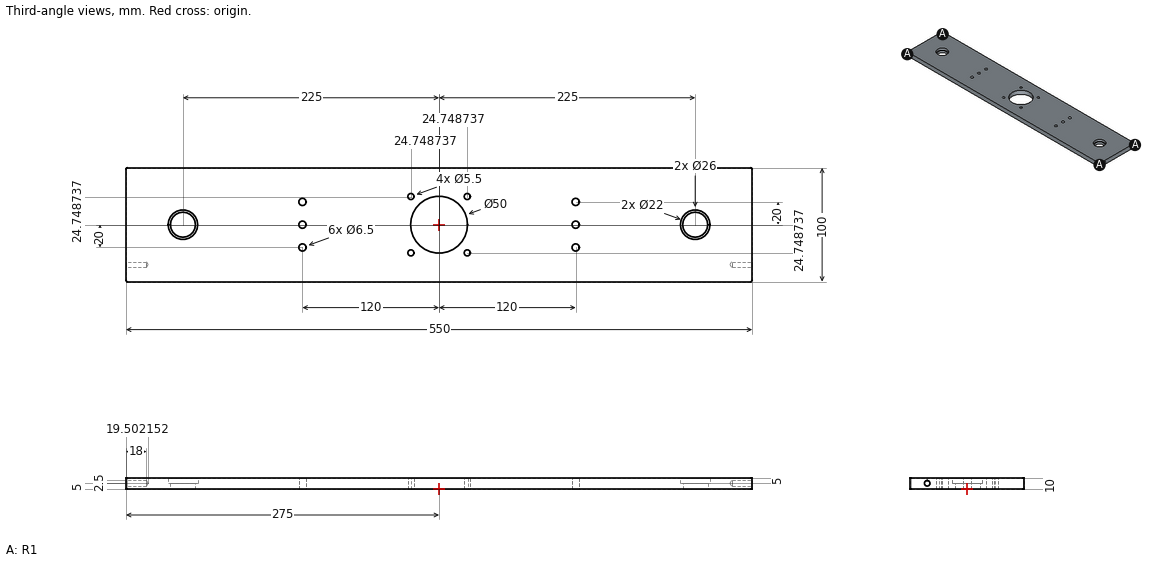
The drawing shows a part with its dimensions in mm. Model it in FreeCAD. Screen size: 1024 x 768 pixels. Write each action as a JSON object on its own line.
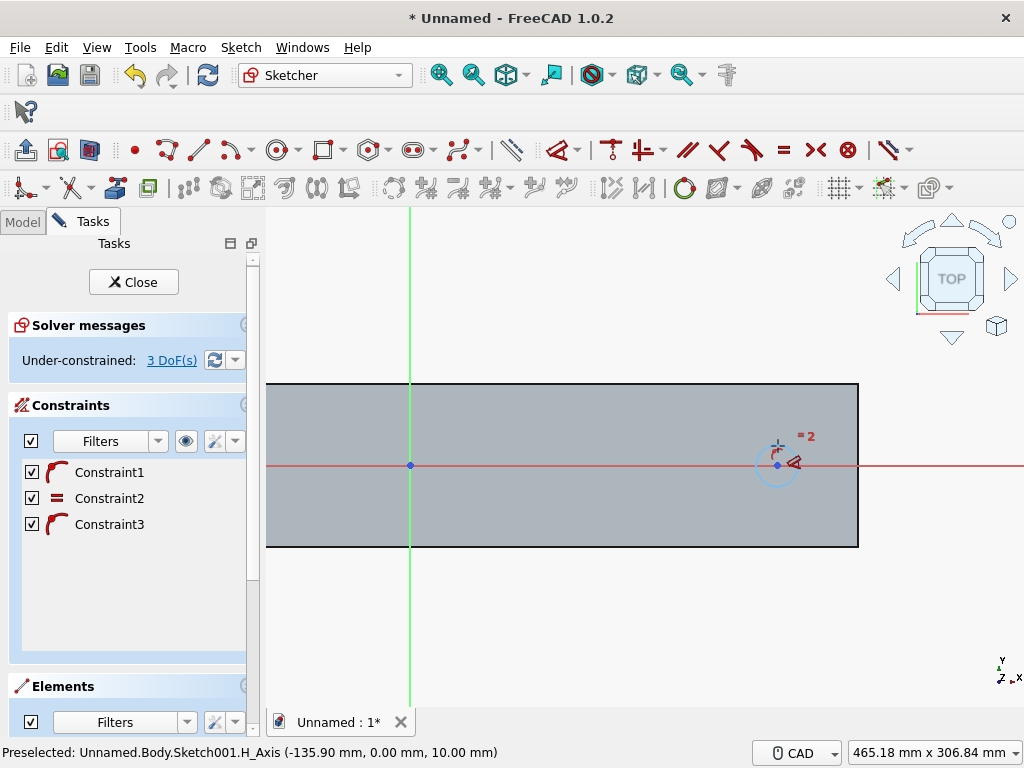
{"action": "left_click", "coordinate": [778, 445]}
{"action": "left_click", "coordinate": [779, 413]}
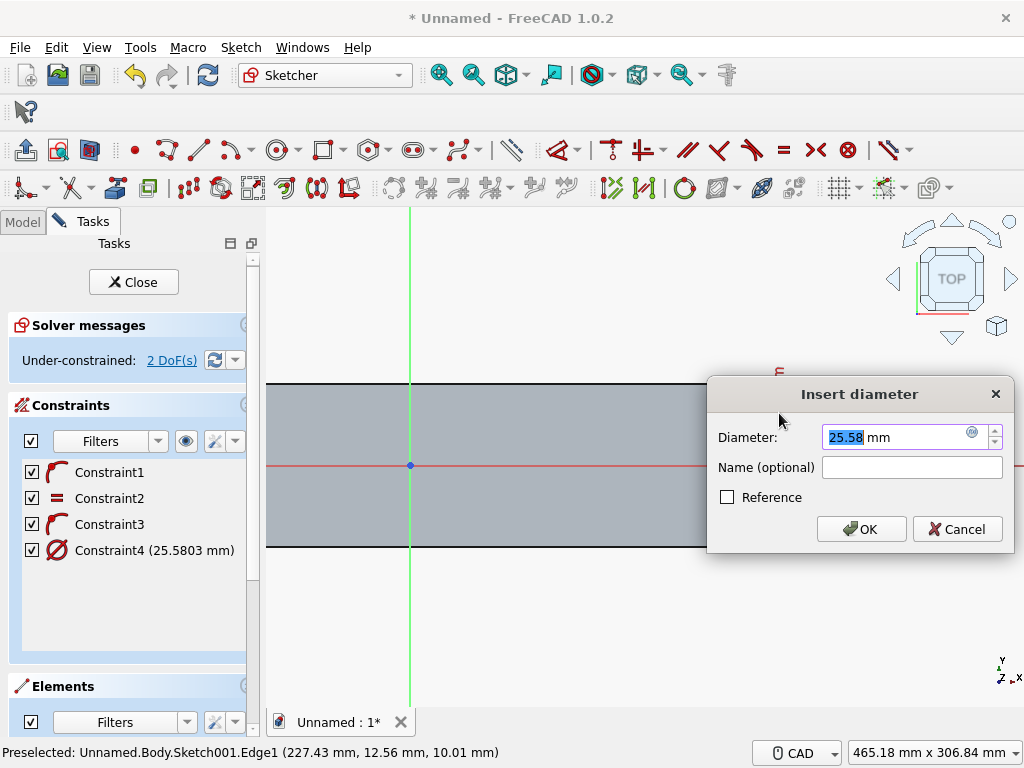
{"action": "type", "text": "26"}
{"action": "key", "text": "Return"}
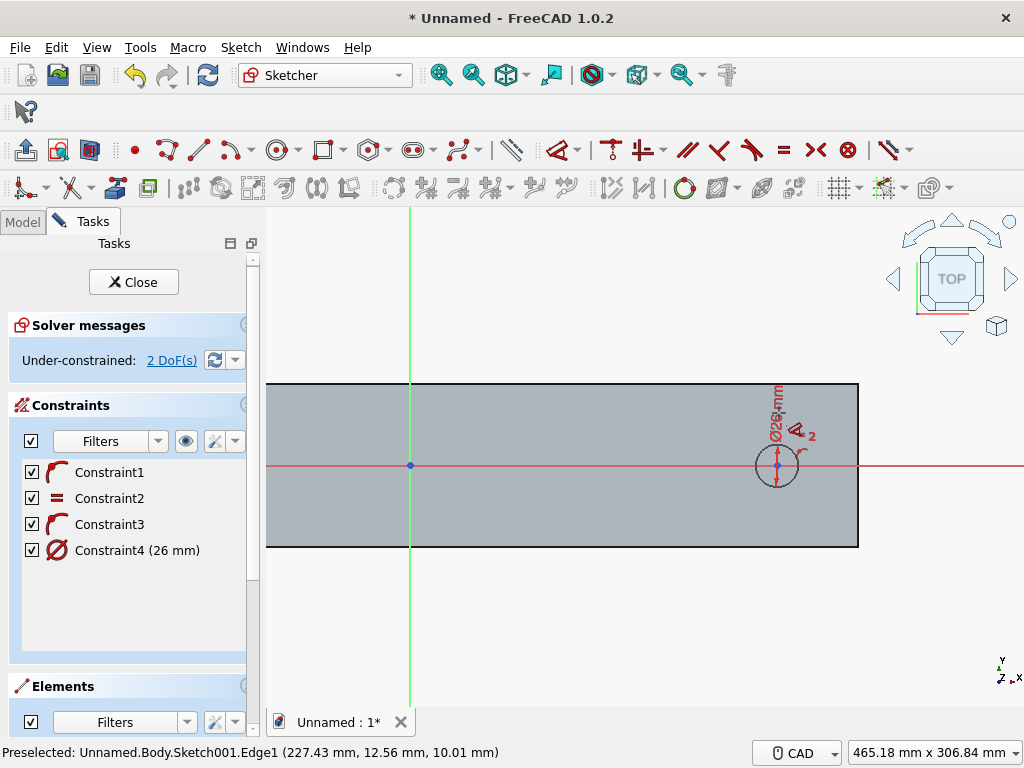
{"action": "left_click", "coordinate": [777, 466]}
{"action": "left_click", "coordinate": [594, 500]}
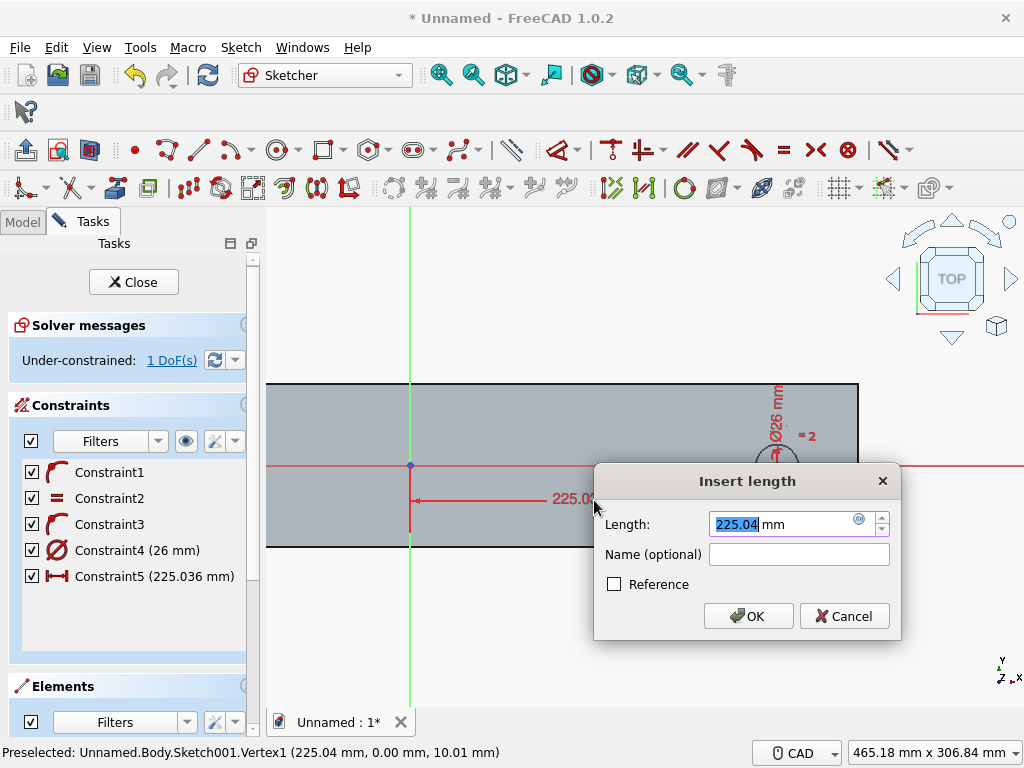
{"action": "type", "text": "225"}
{"action": "key", "text": "Return"}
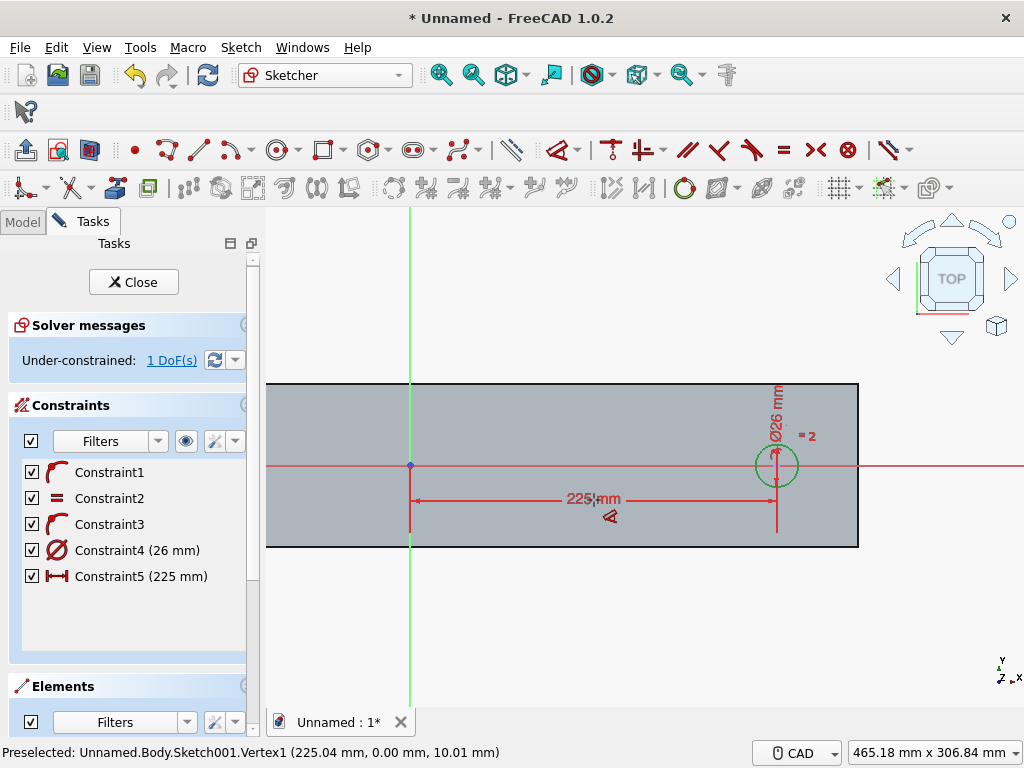
{"action": "scroll", "coordinate": [779, 446], "scroll_direction": "down", "scroll_amount": 3}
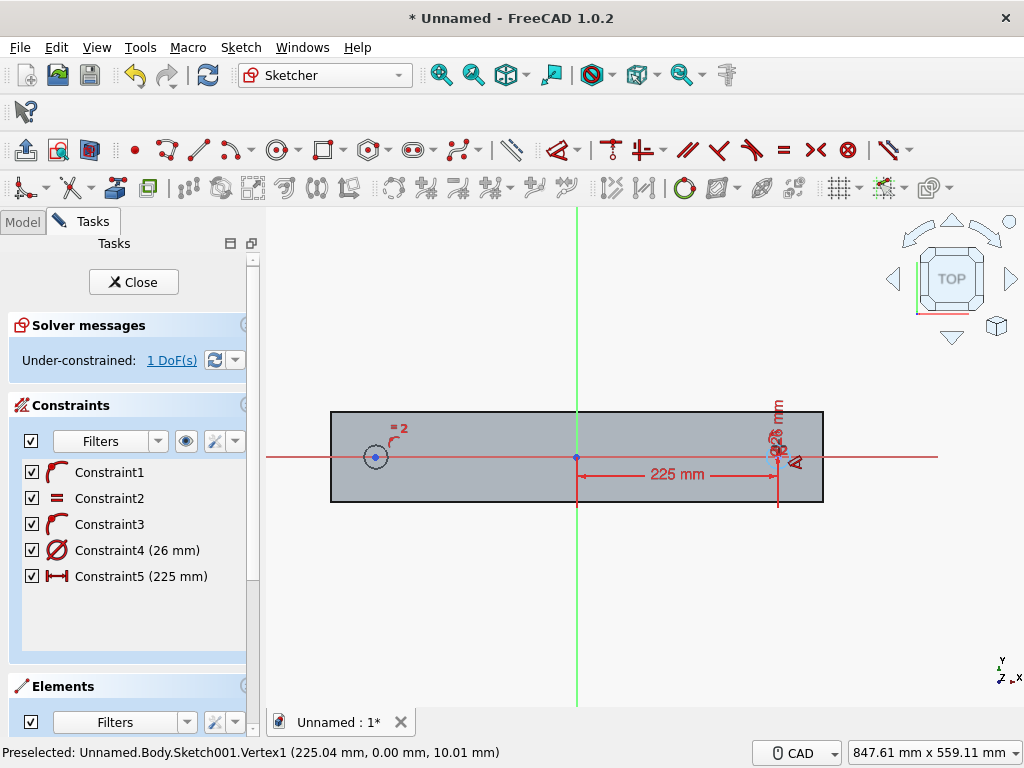
{"action": "left_click", "coordinate": [376, 457]}
{"action": "left_click", "coordinate": [476, 491]}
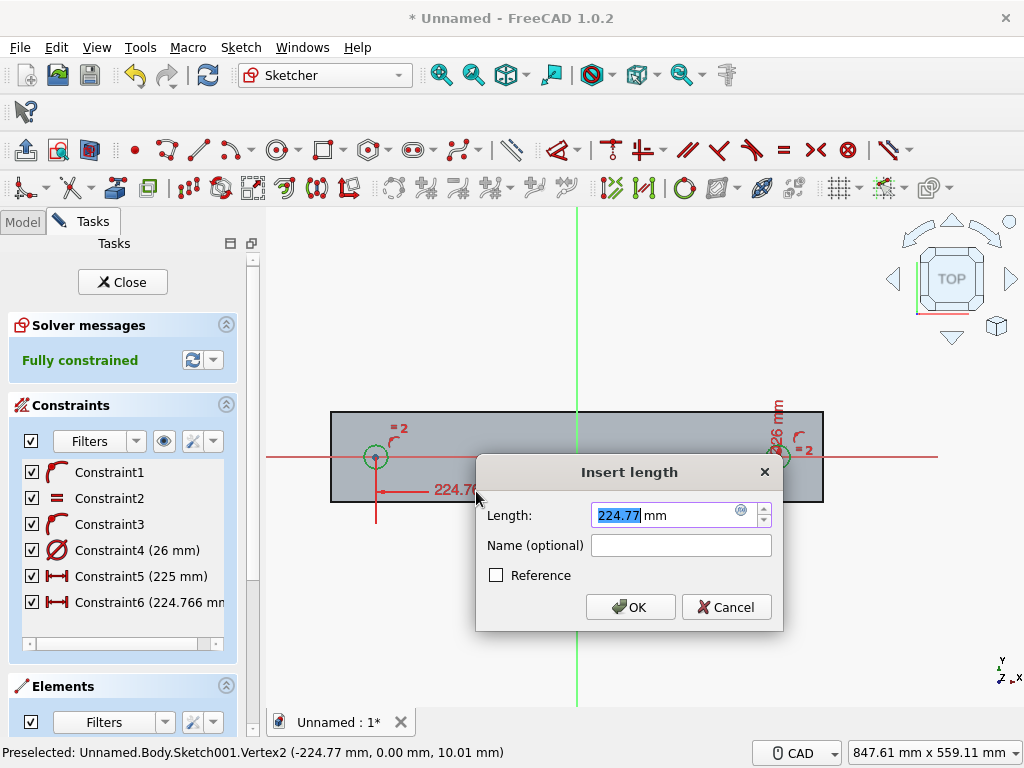
{"action": "type", "text": "225"}
{"action": "key", "text": "Return"}
{"action": "key", "text": "Escape"}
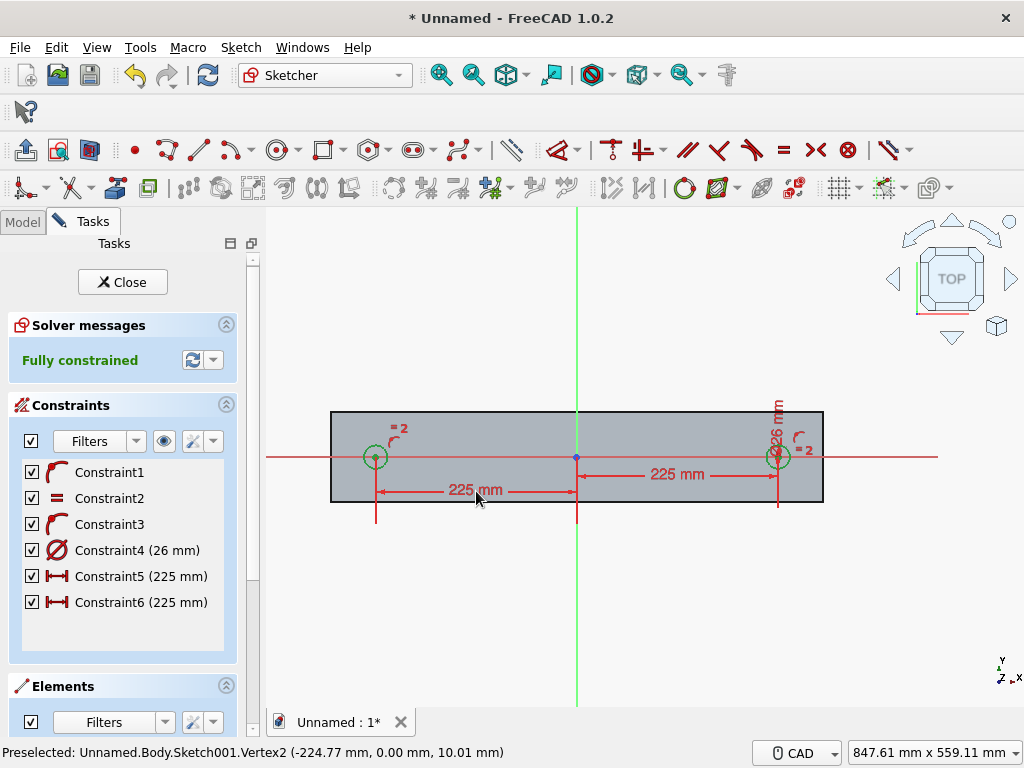
{"action": "left_click", "coordinate": [123, 282]}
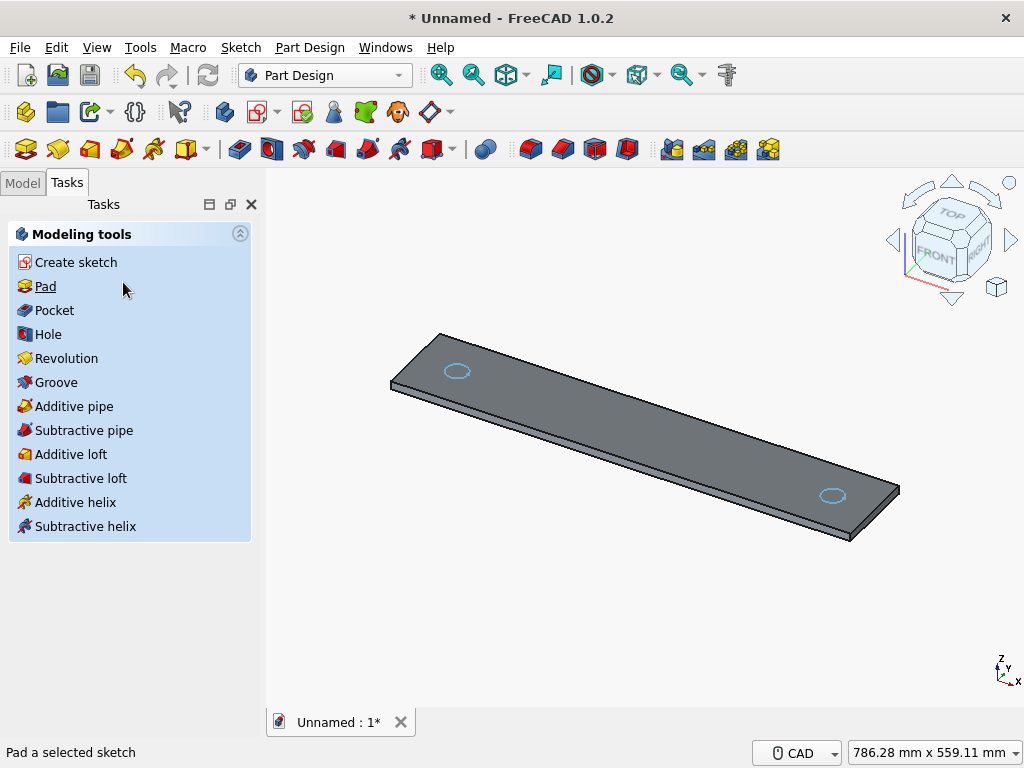
{"action": "left_click", "coordinate": [240, 150]}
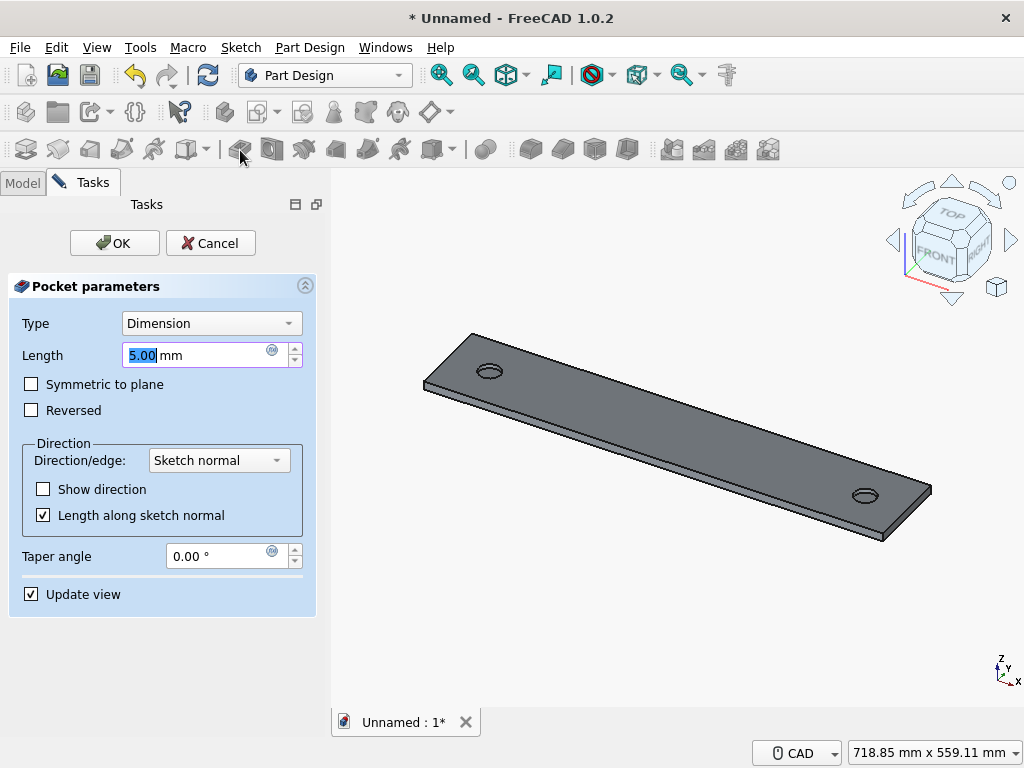
{"action": "type", "text": "5"}
{"action": "key", "text": "Tab"}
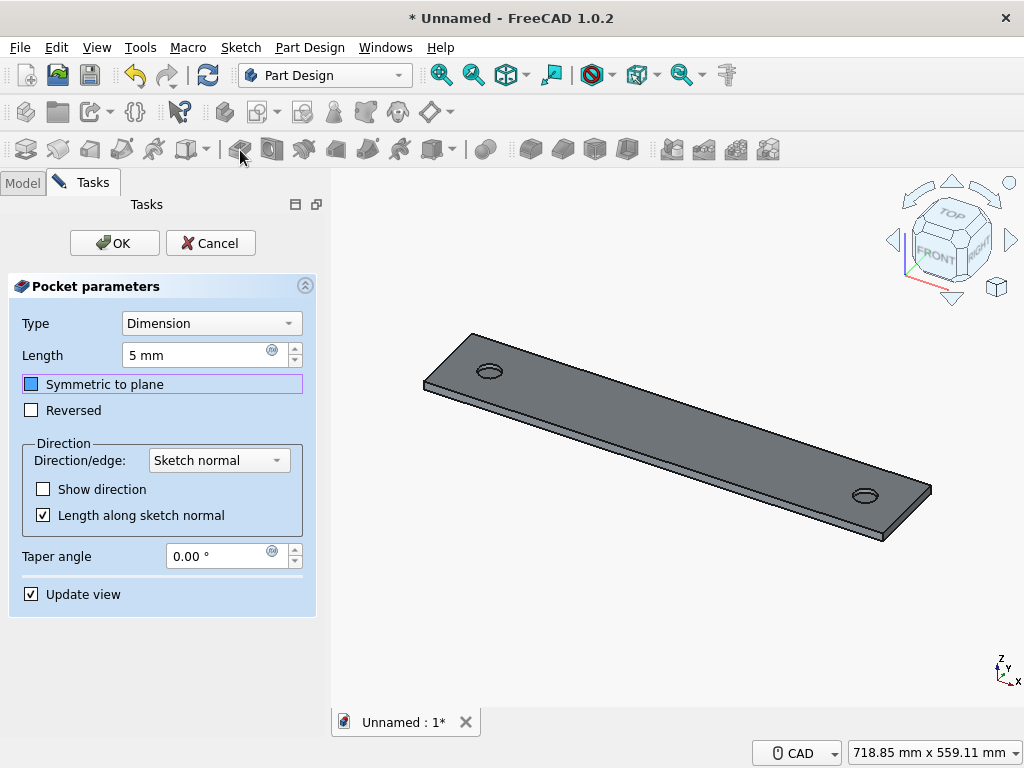
{"action": "left_click", "coordinate": [115, 243]}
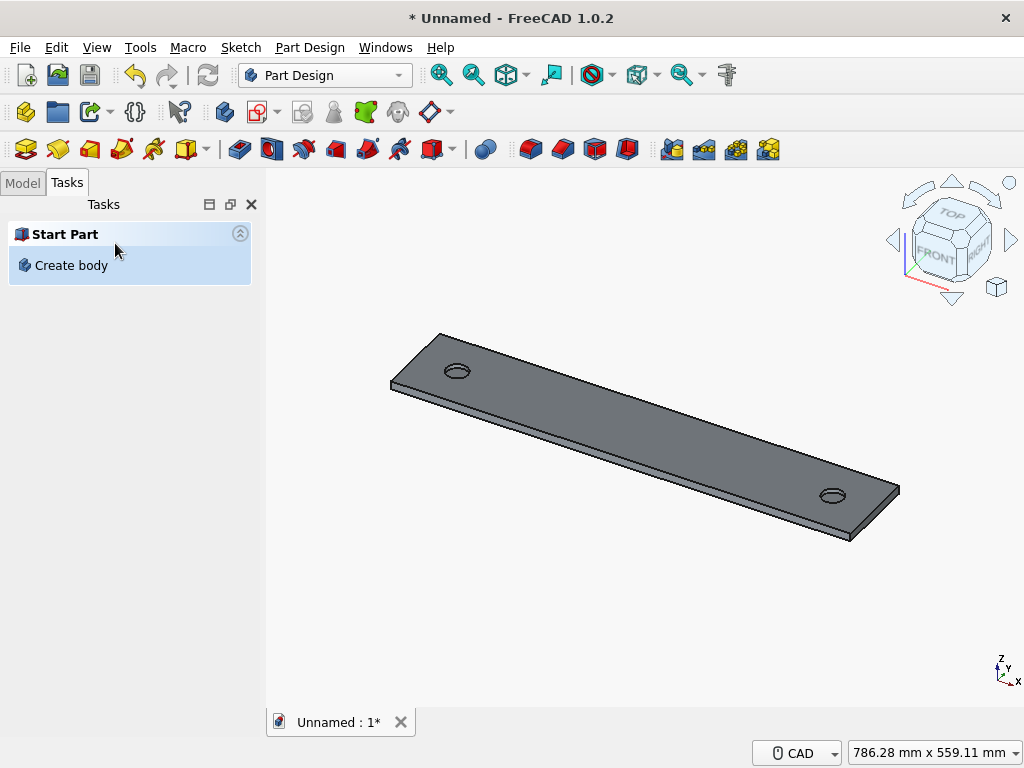
{"action": "key", "text": "0"}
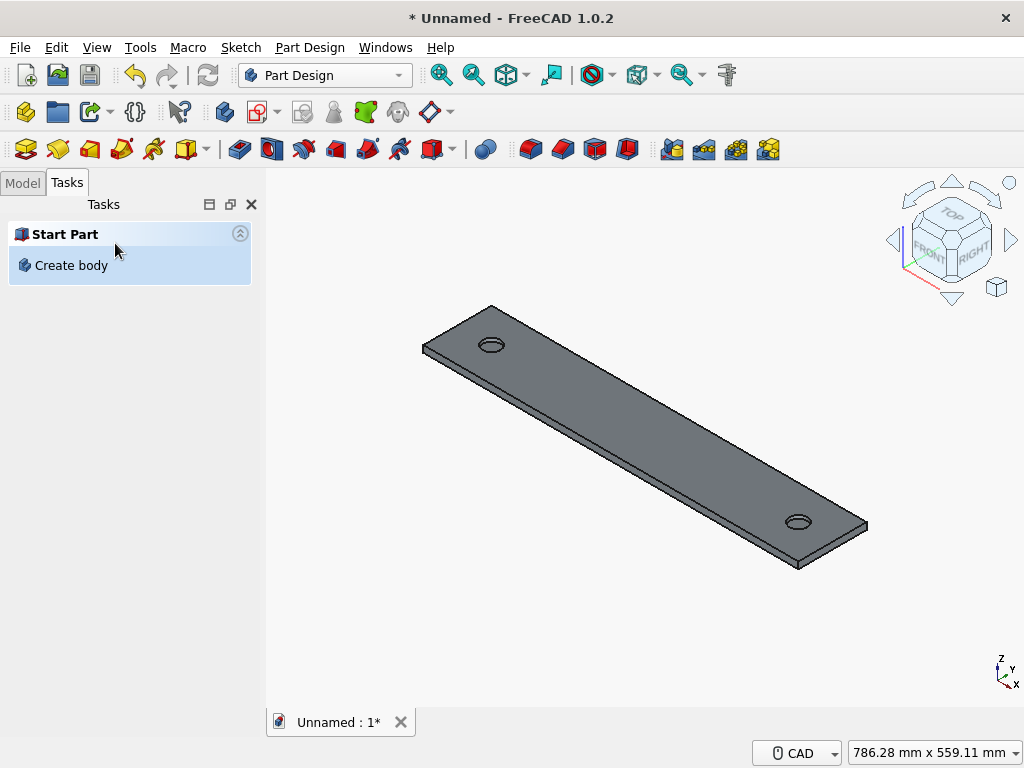
{"action": "key", "text": "2"}